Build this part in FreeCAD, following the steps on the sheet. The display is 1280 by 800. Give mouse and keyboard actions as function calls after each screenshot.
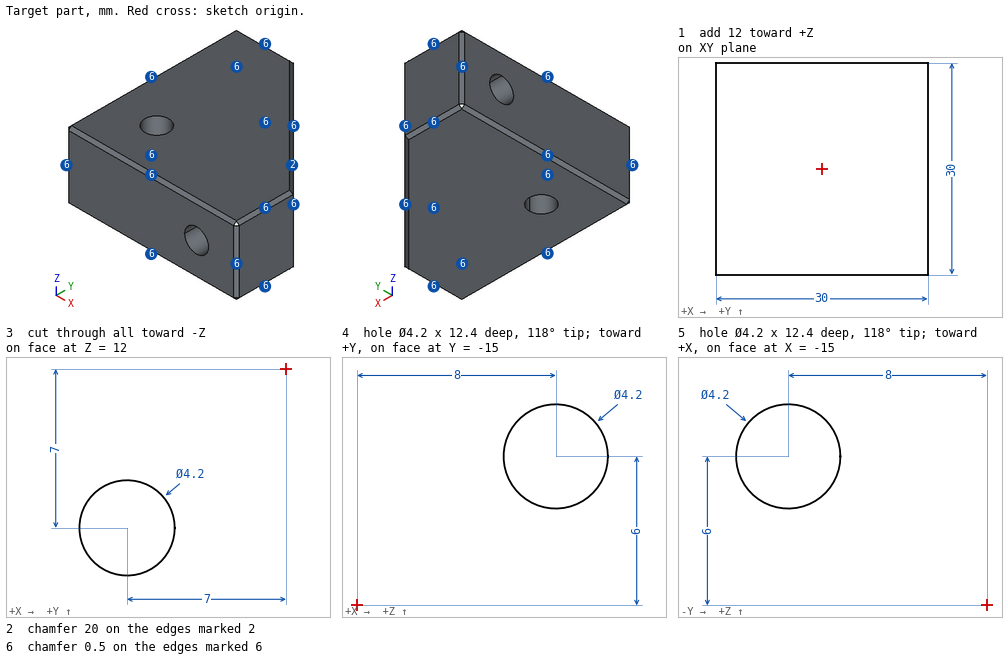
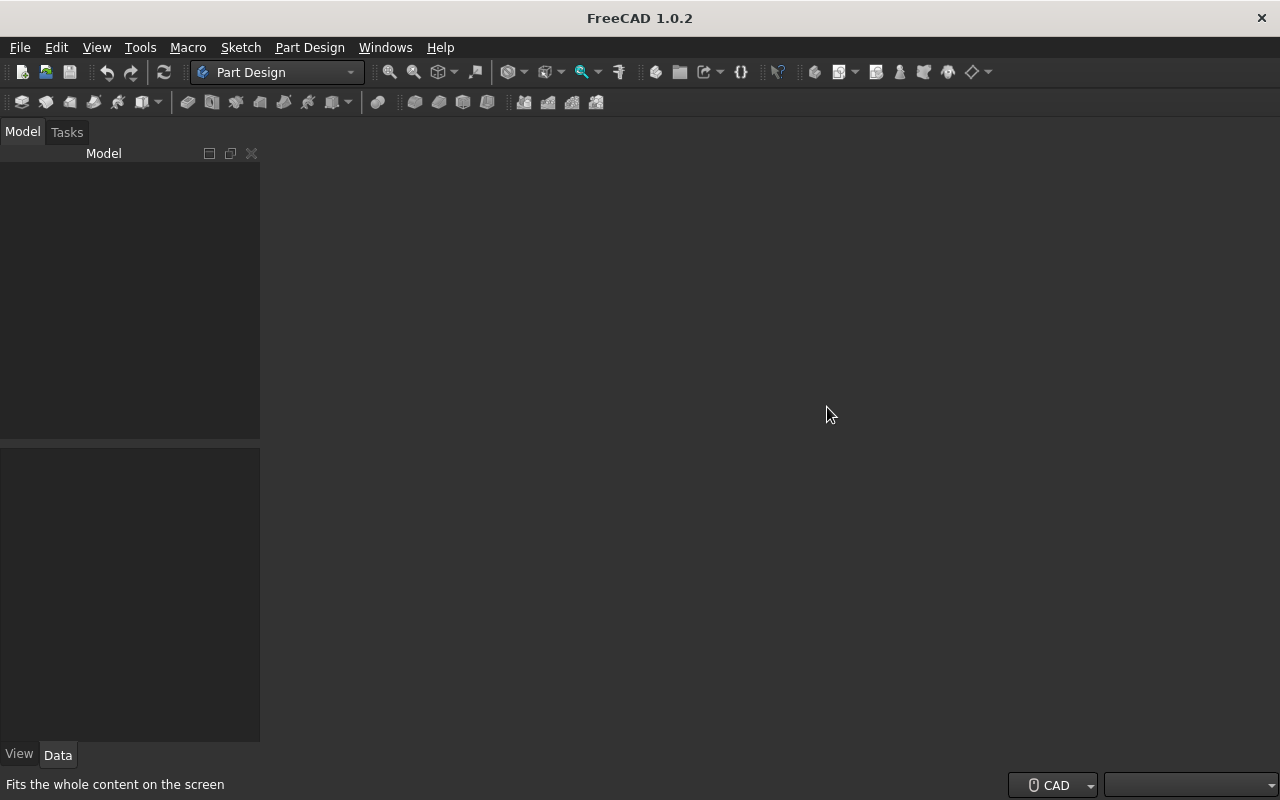
click(22, 72)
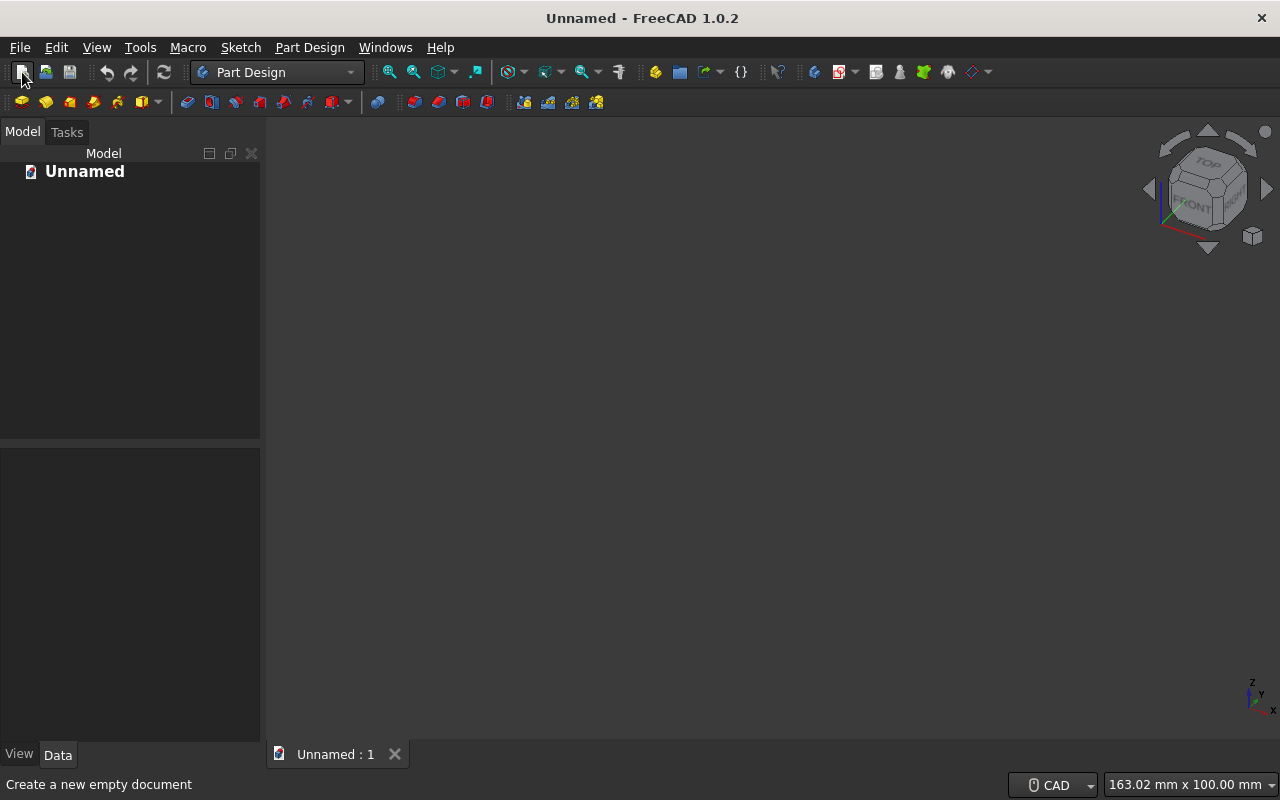
click(840, 72)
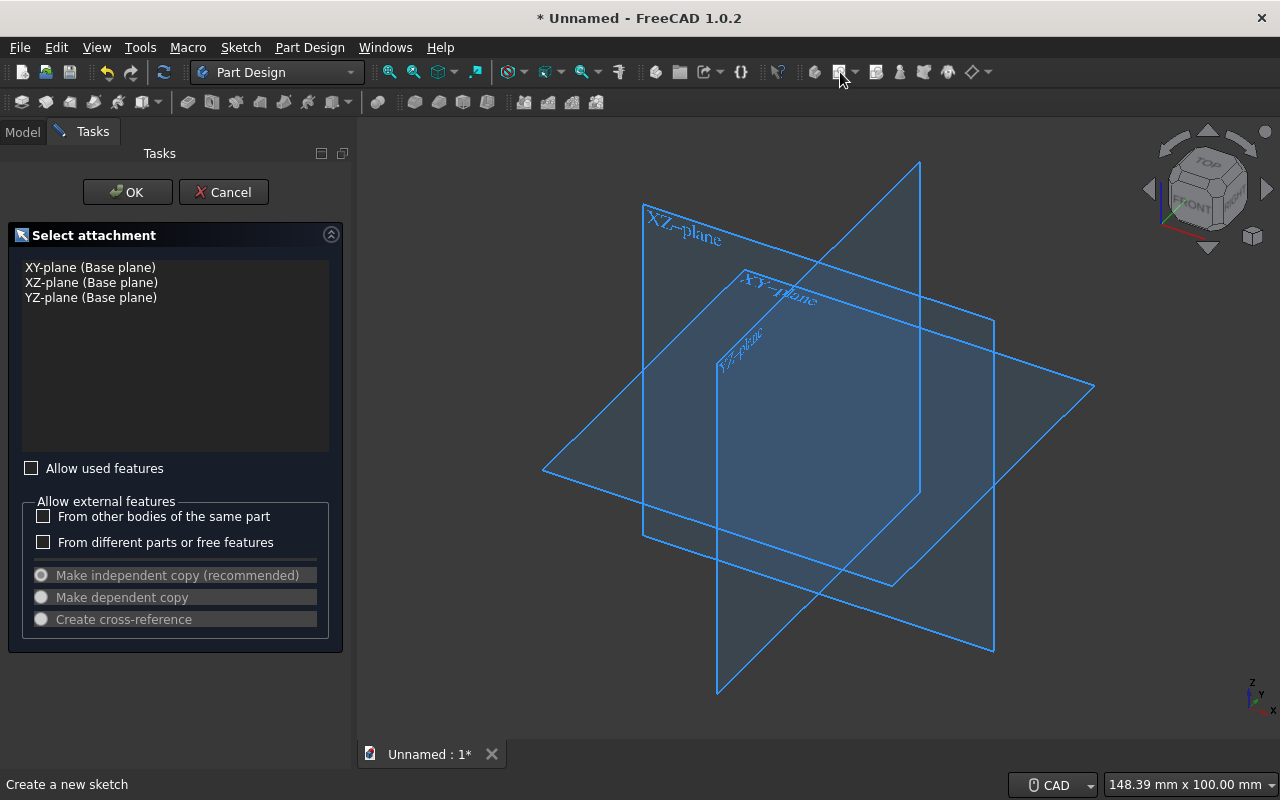
click(82, 268)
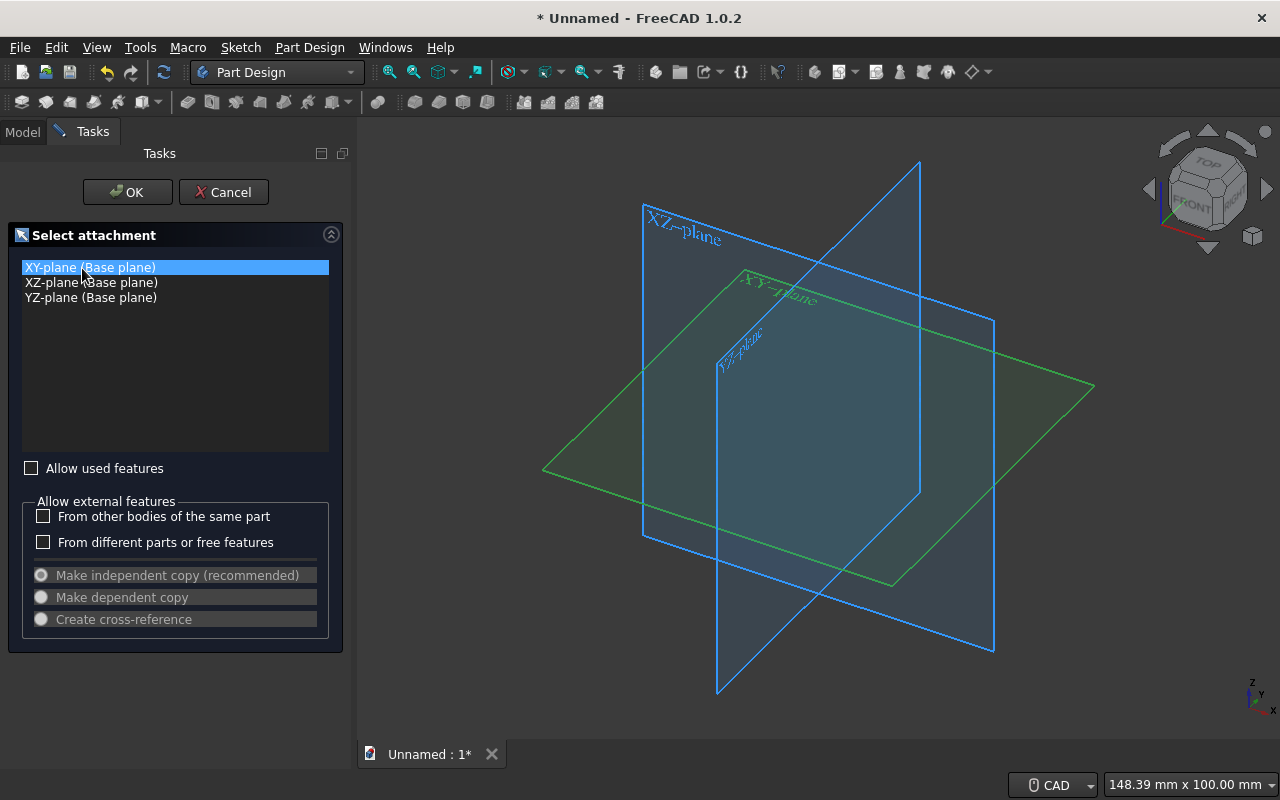
click(128, 192)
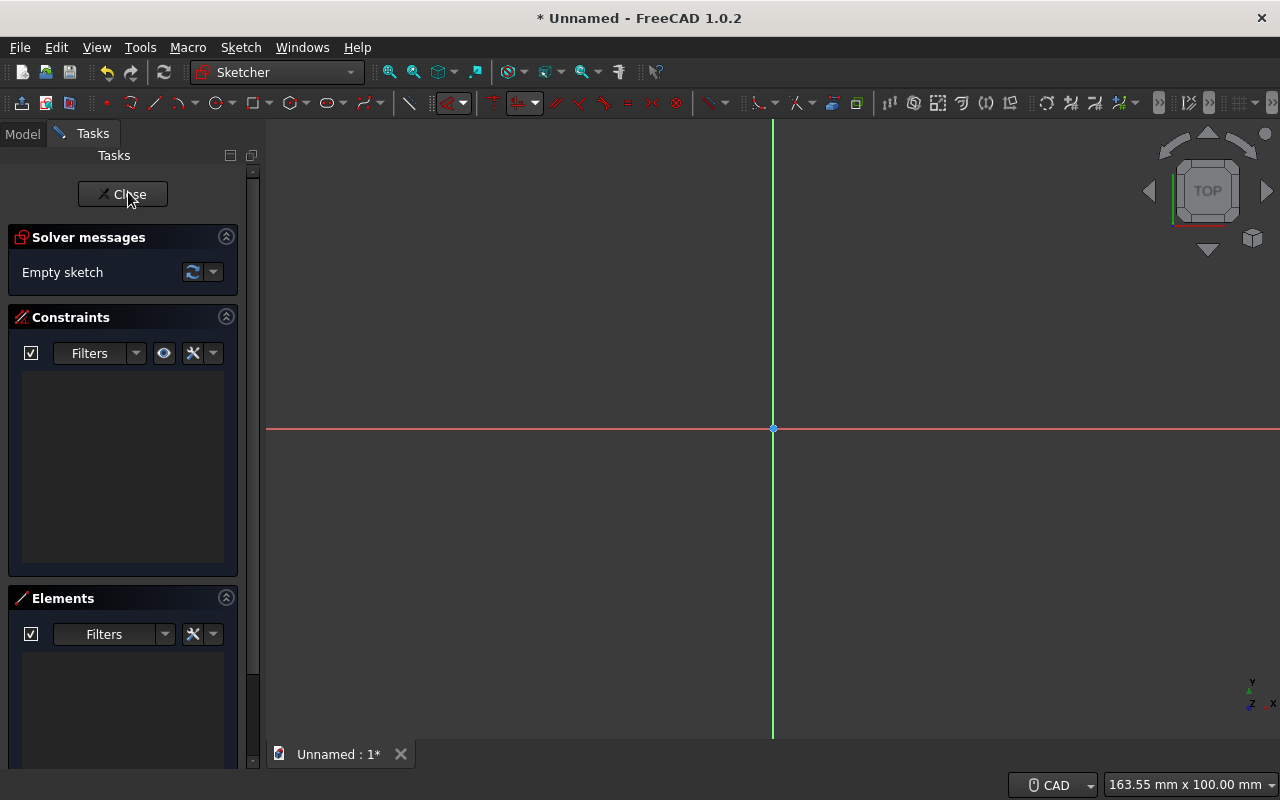
scroll(829, 429, up, 4)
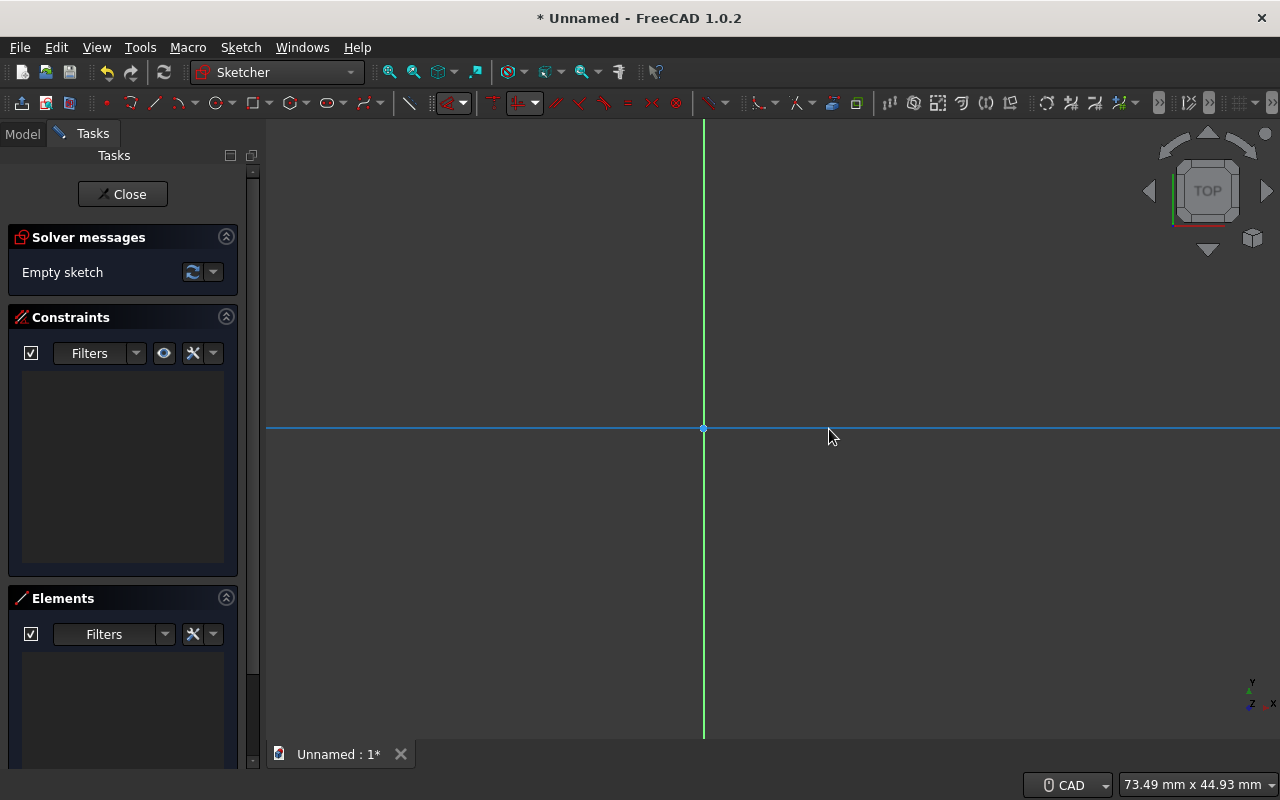
key(g)
key(v)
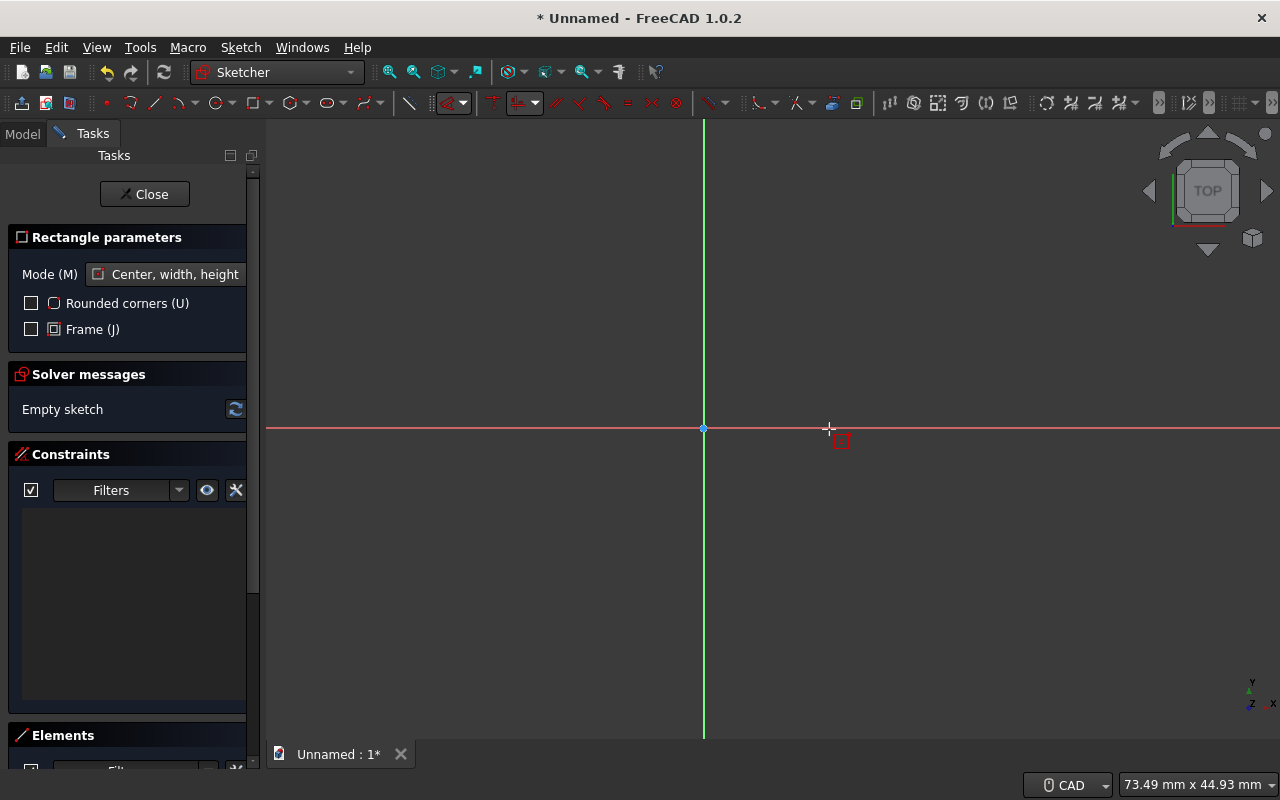
click(704, 428)
click(911, 221)
key(Escape)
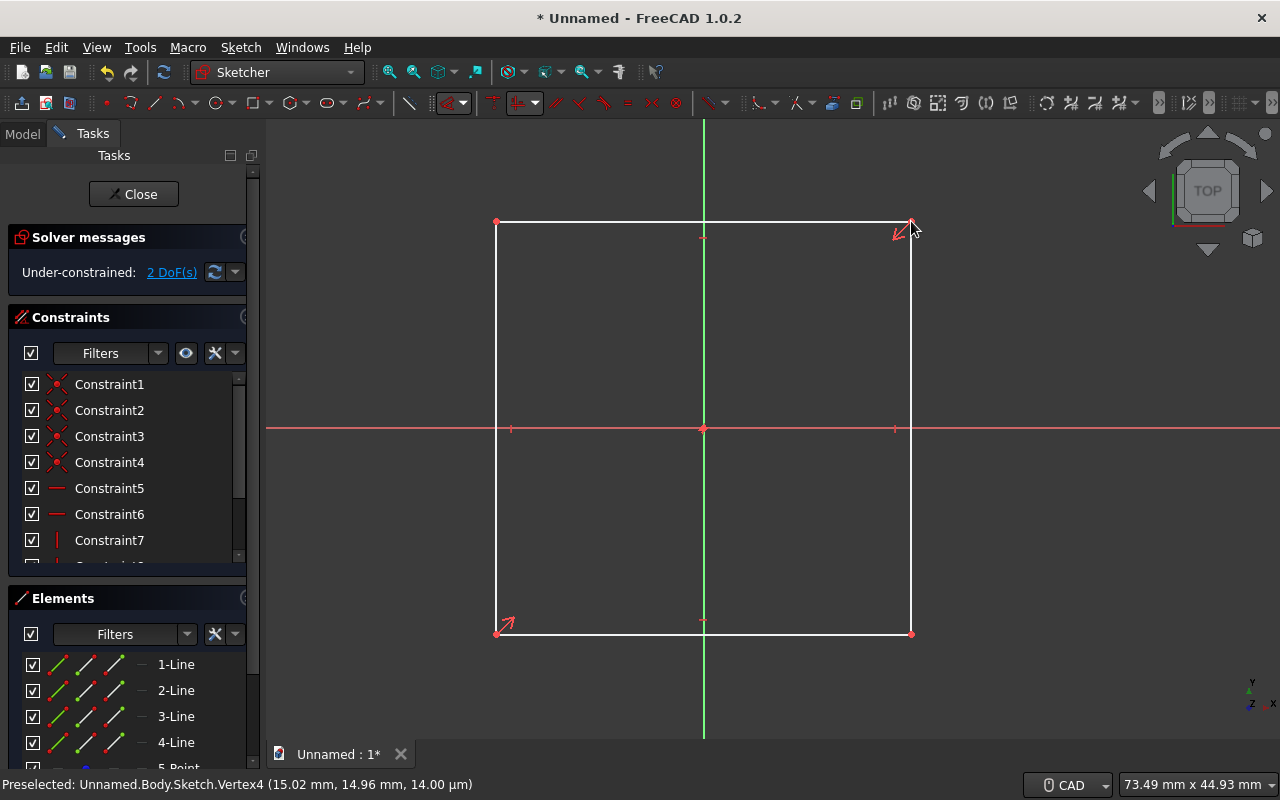
key(d)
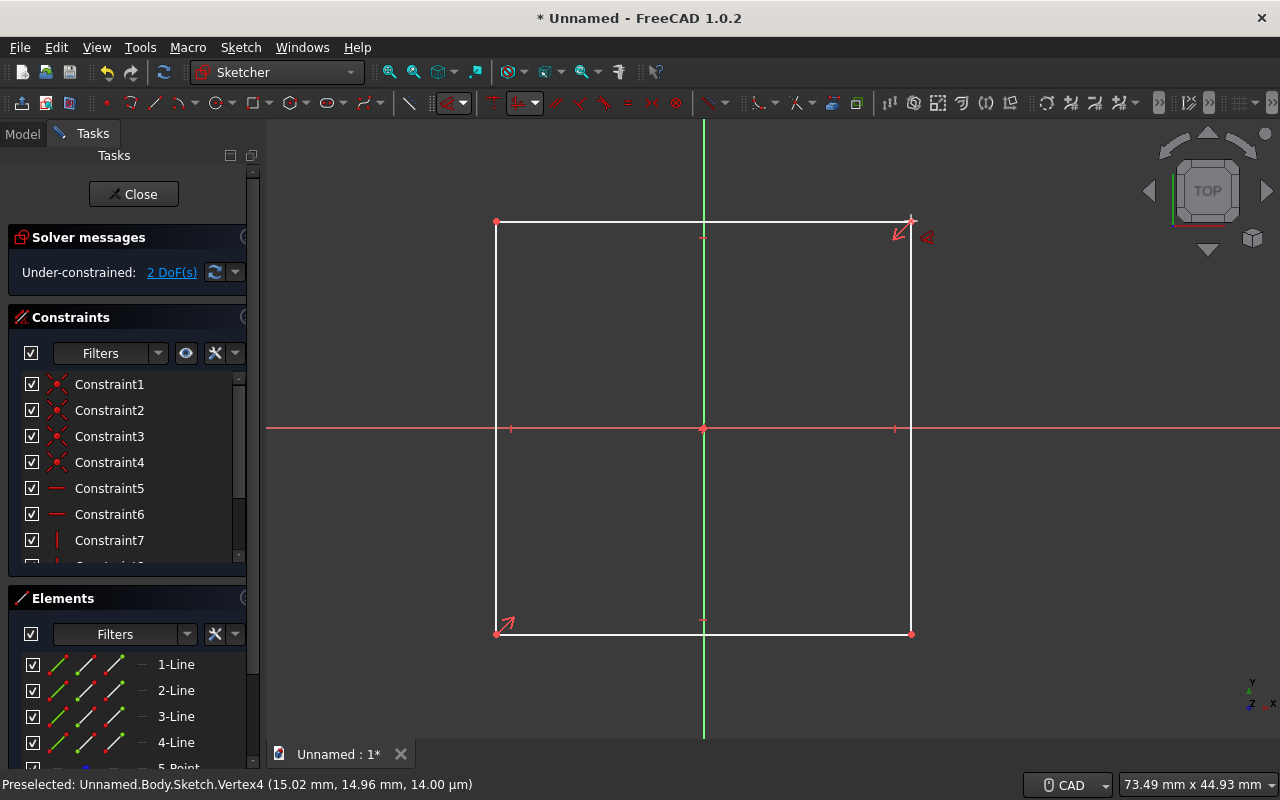
click(621, 635)
click(608, 669)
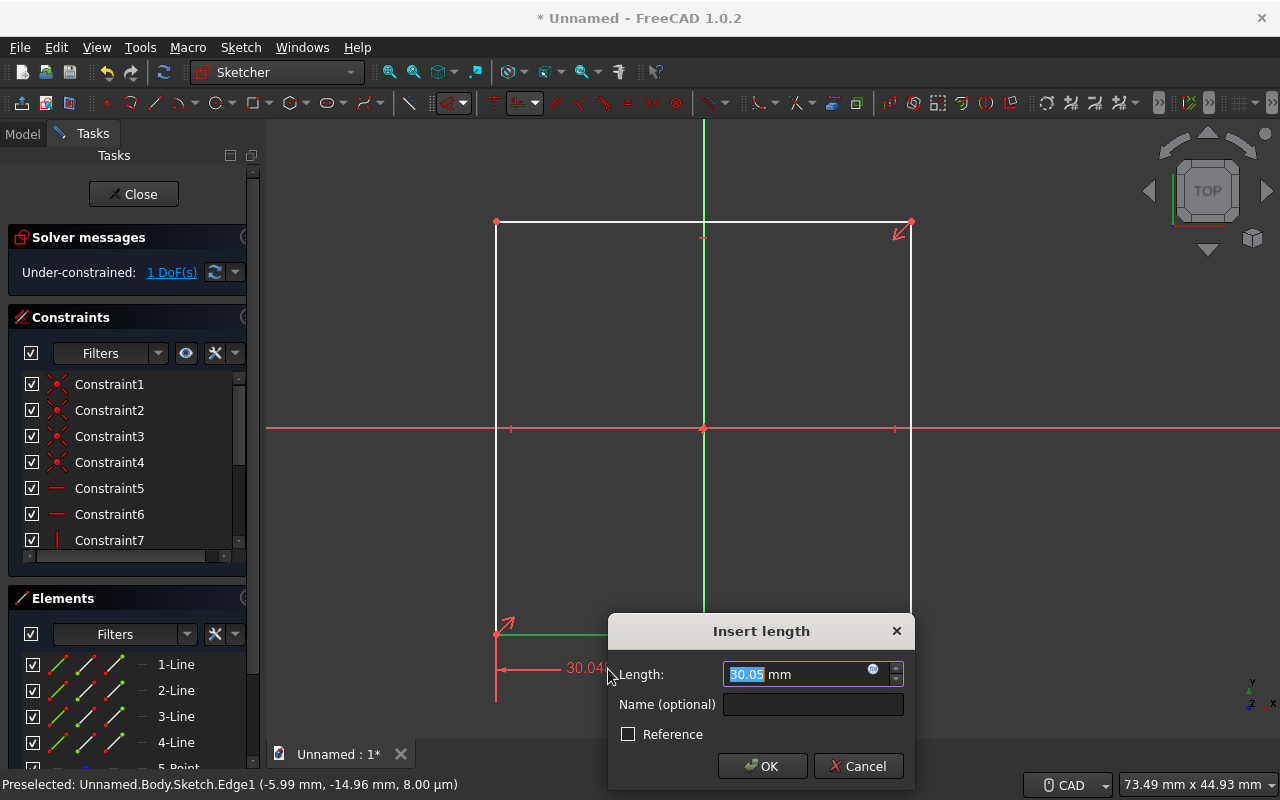
text(30)
key(Return)